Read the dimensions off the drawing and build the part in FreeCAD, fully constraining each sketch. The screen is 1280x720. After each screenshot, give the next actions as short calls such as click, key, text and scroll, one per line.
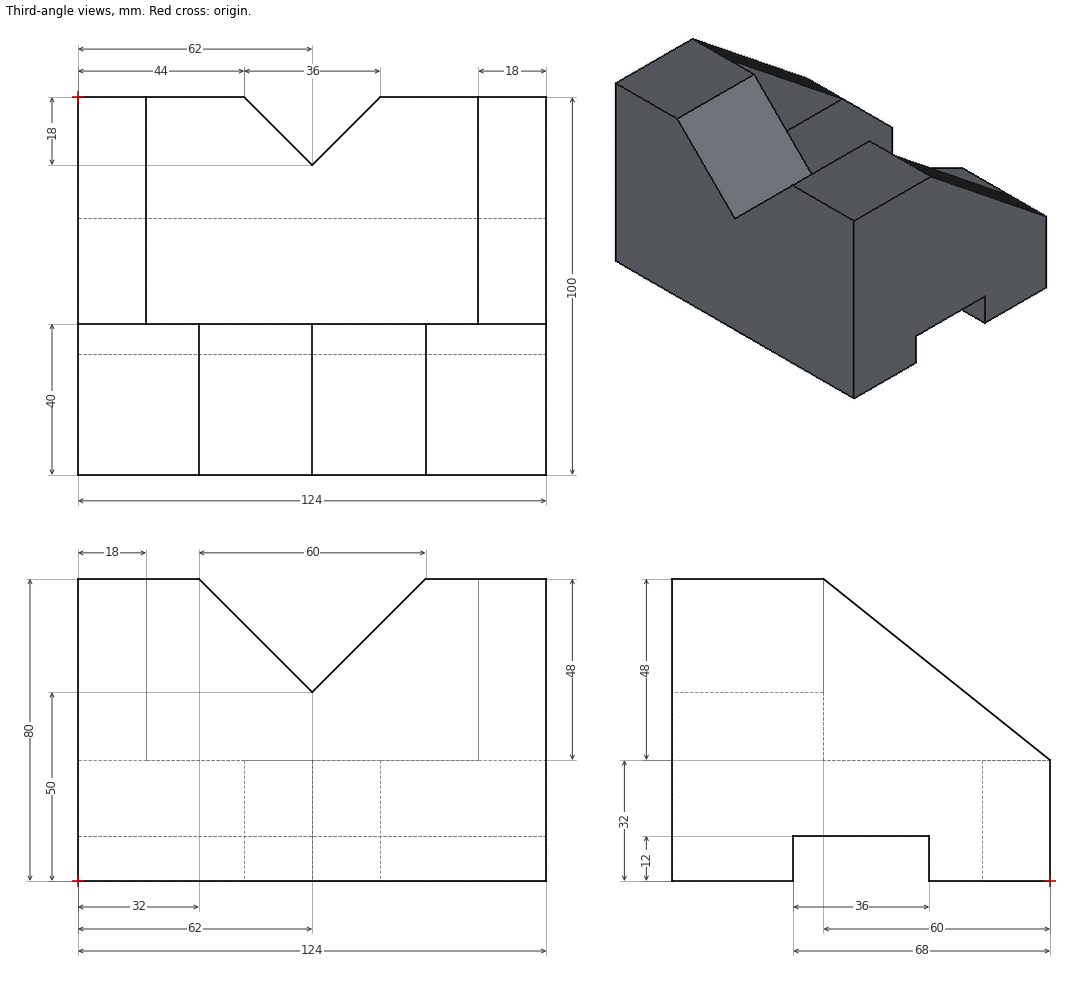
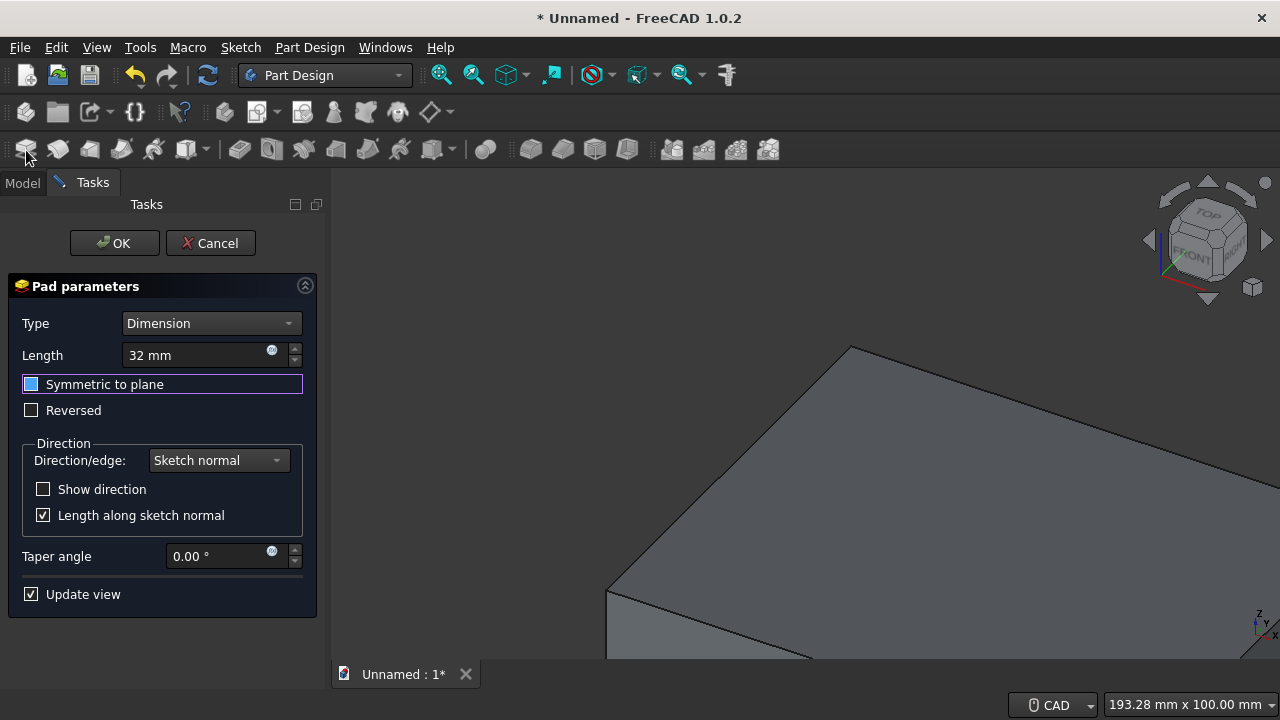
click(115, 243)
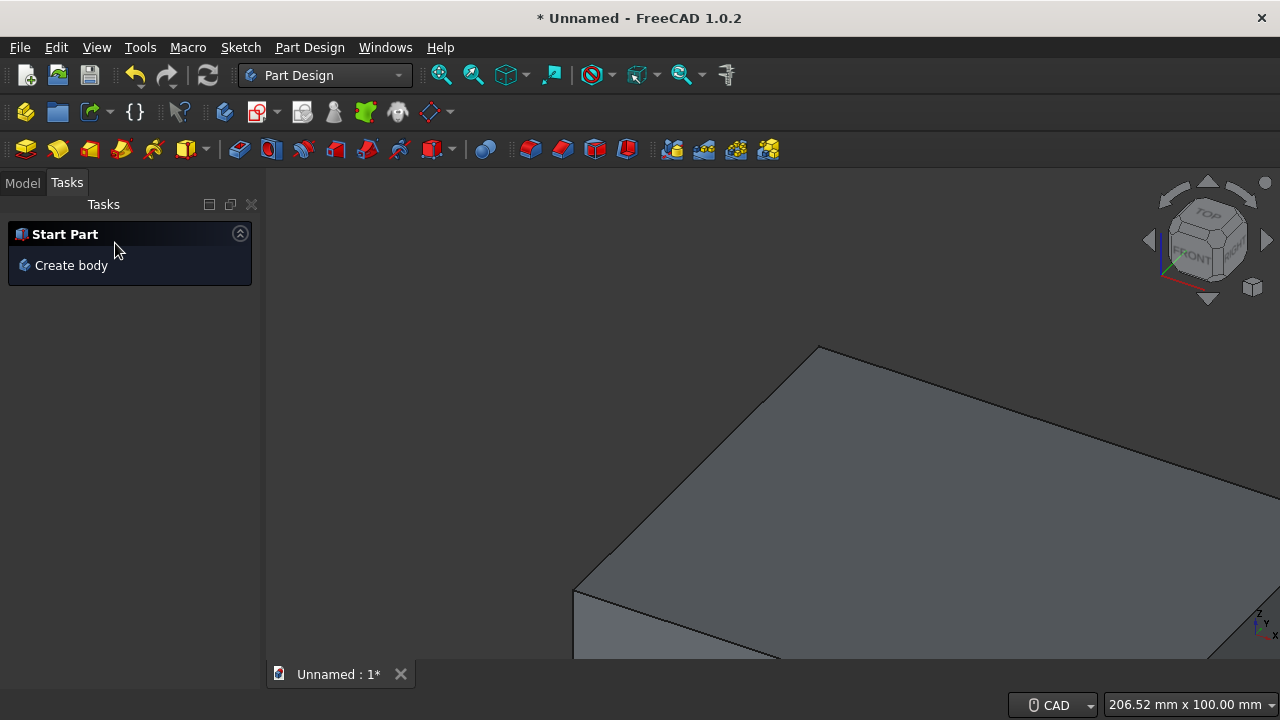
click(442, 76)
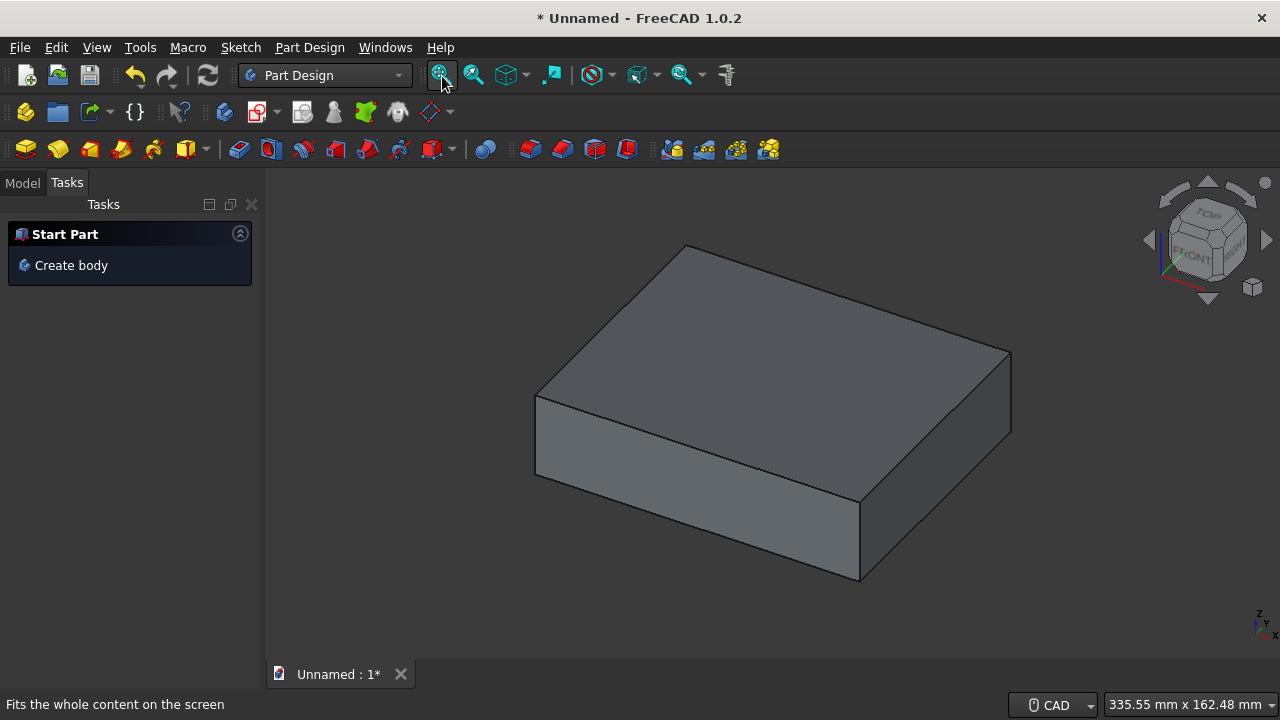
click(258, 112)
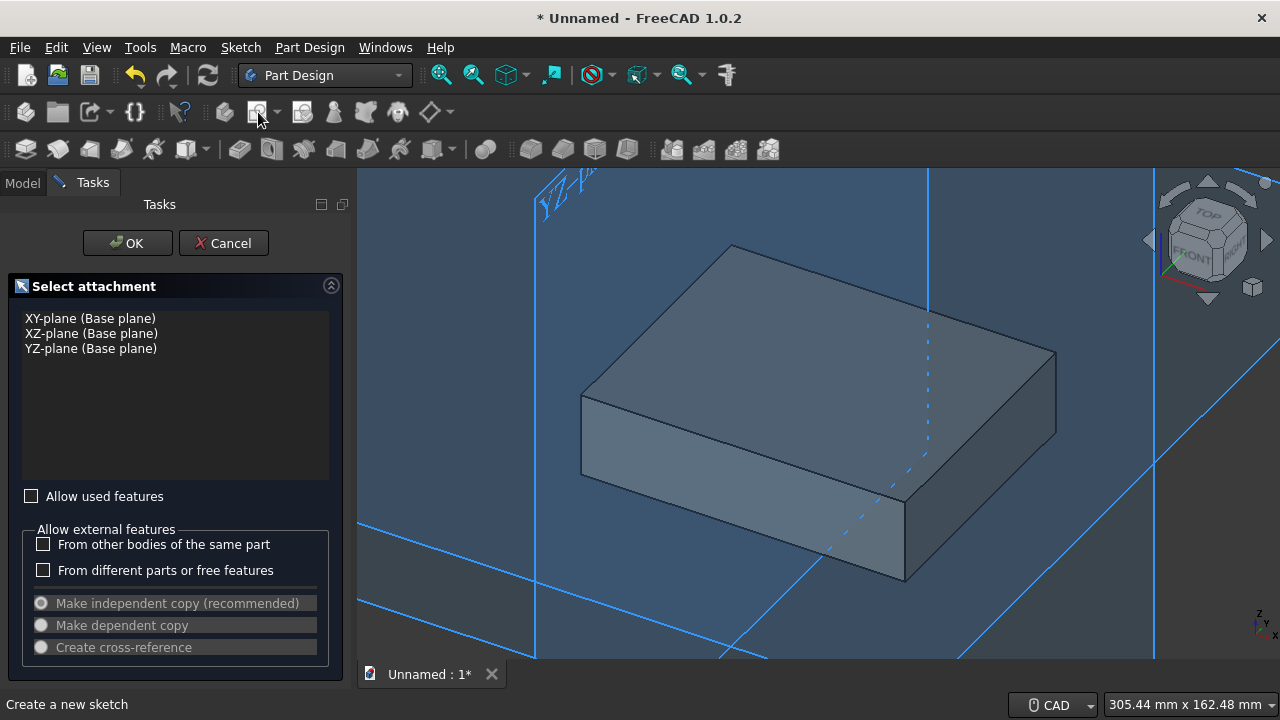
click(82, 348)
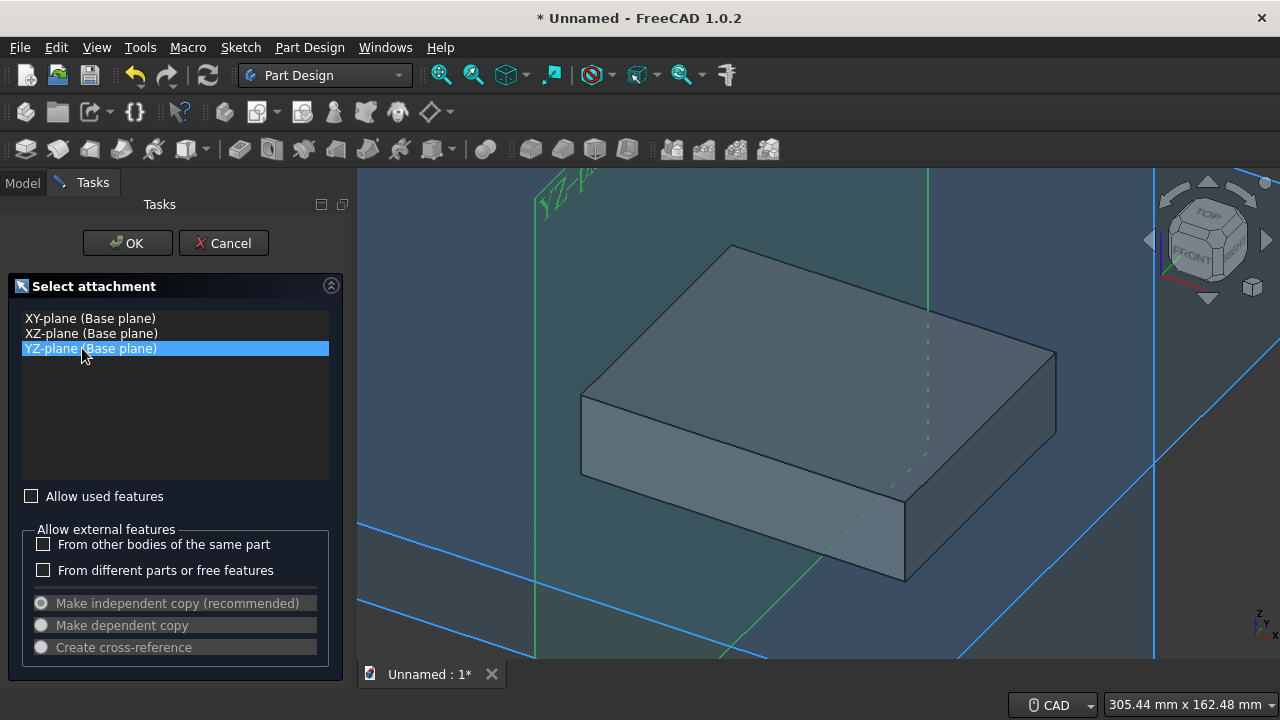
click(128, 243)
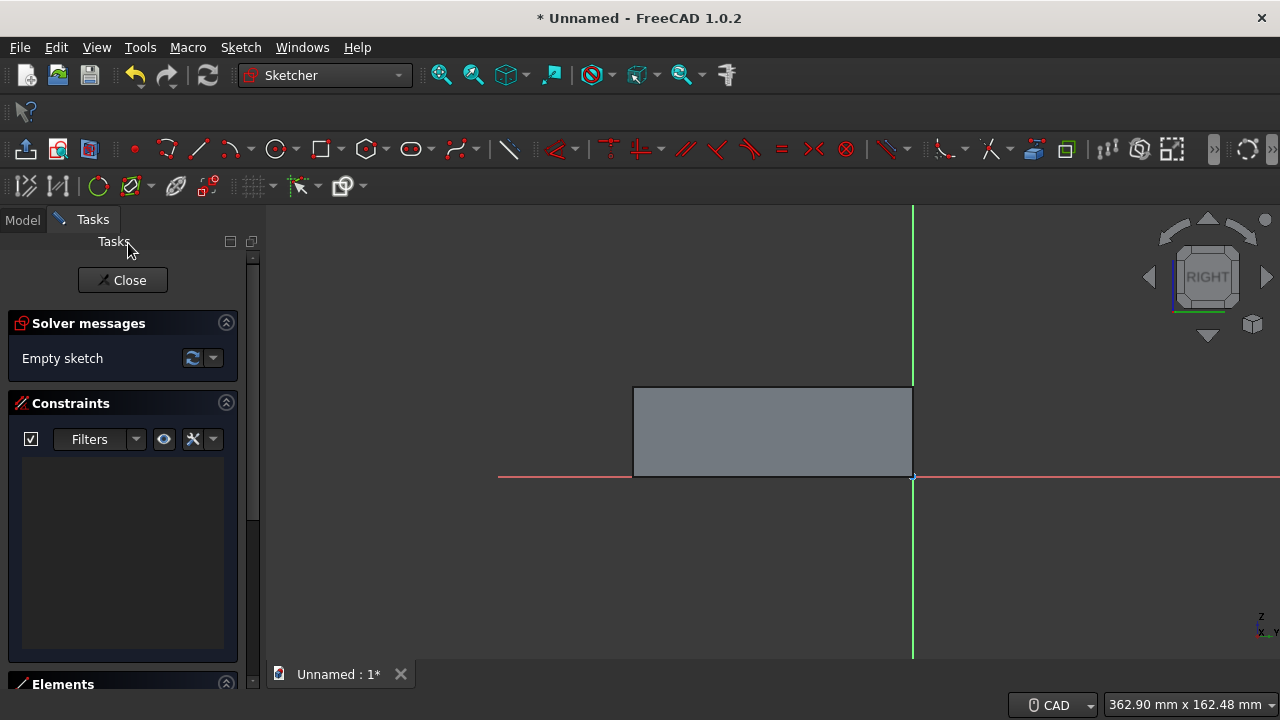
click(90, 150)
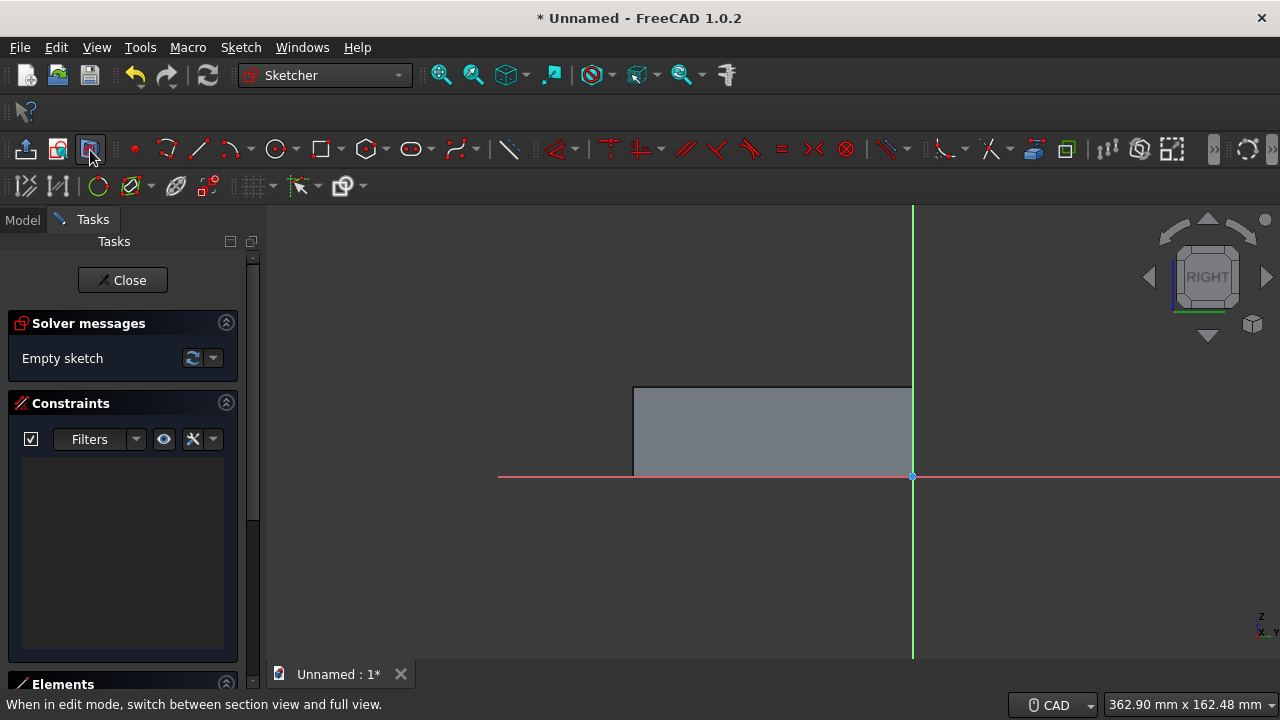
scroll(867, 472, up, 6)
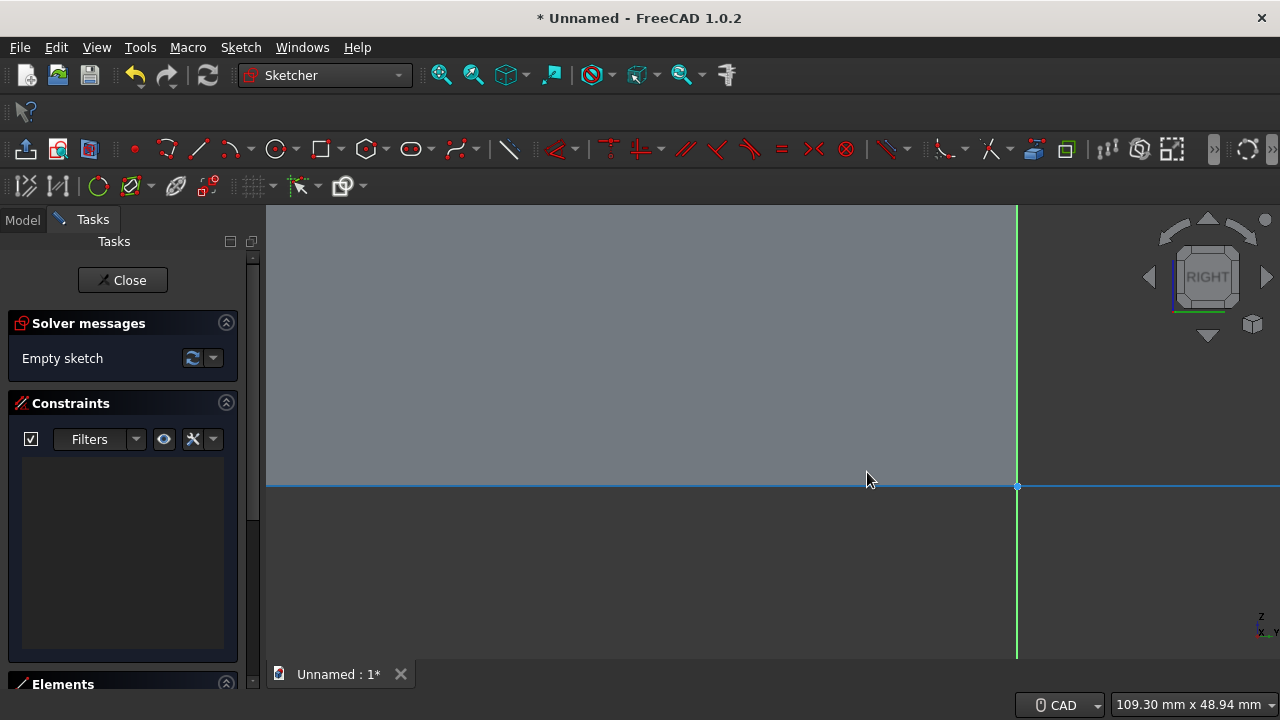
click(322, 150)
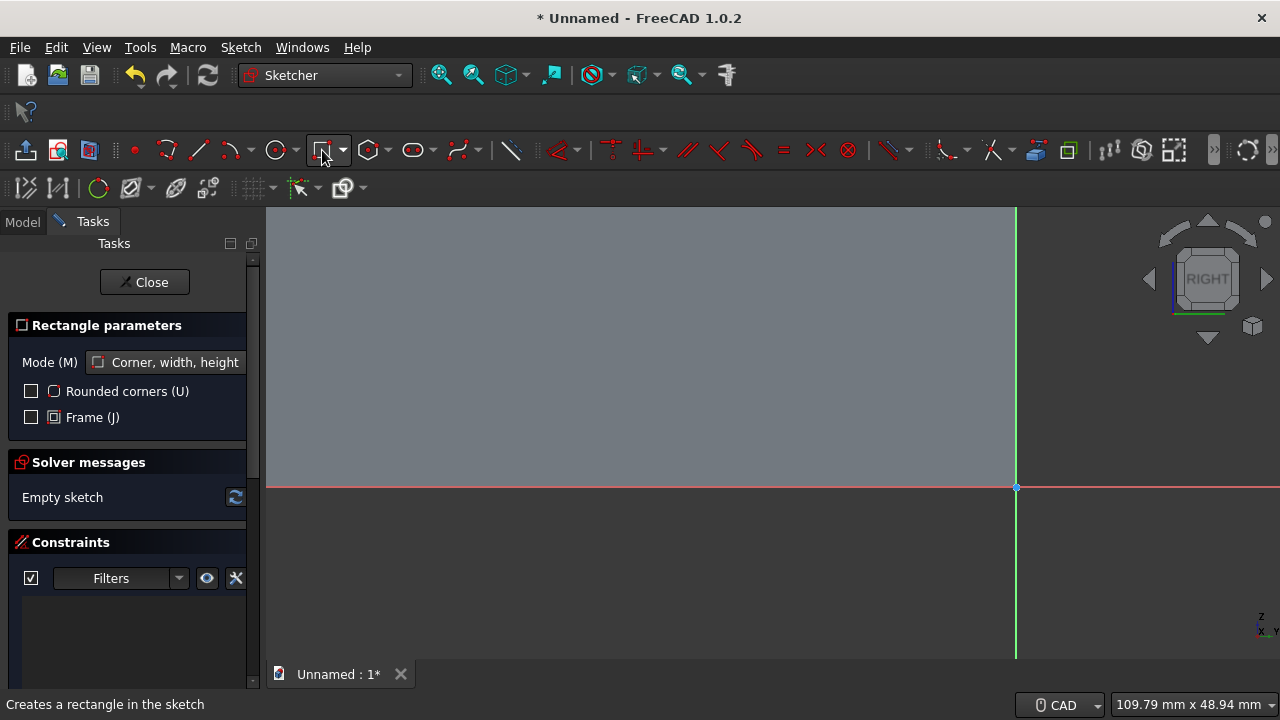
click(388, 376)
click(721, 487)
key(Escape)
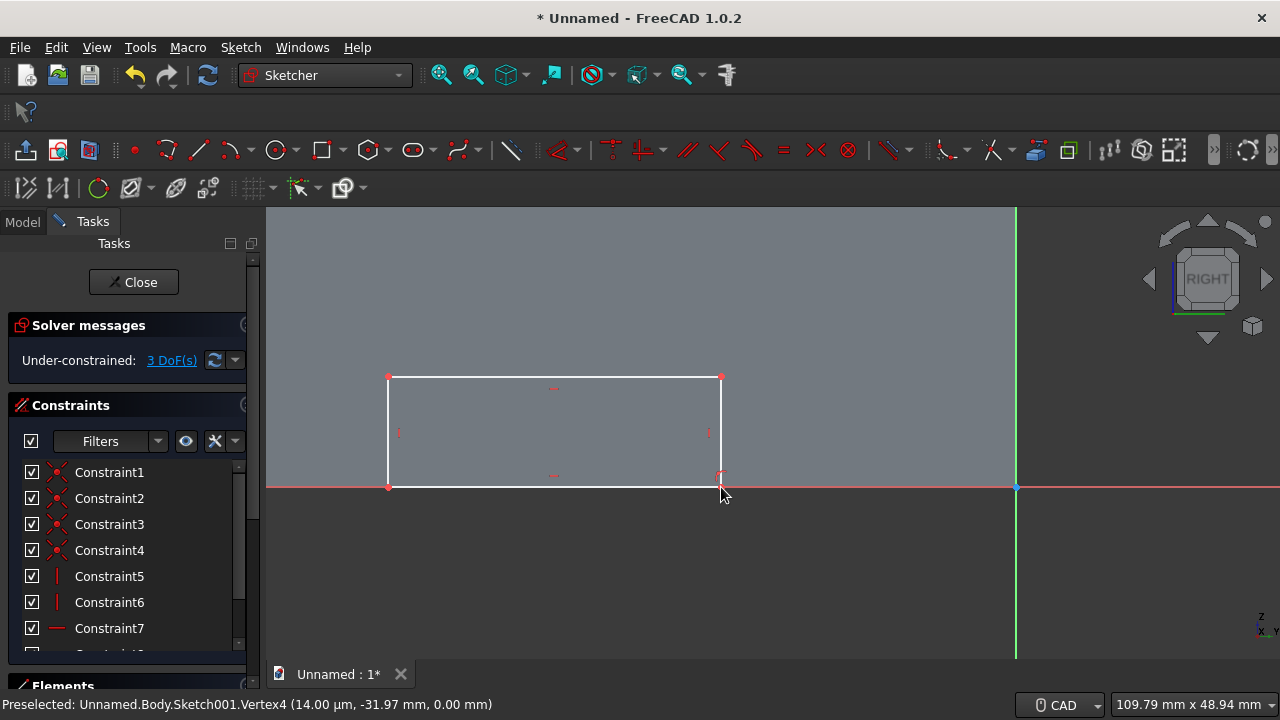
click(558, 150)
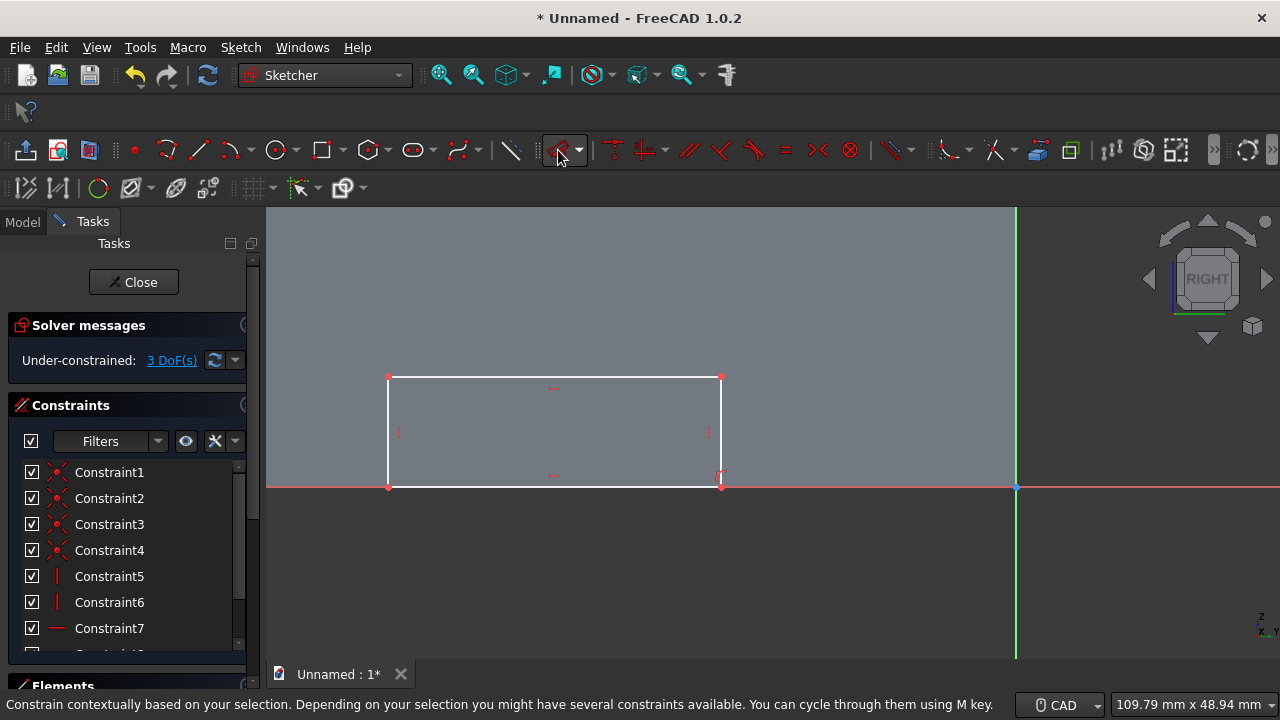
click(388, 410)
click(354, 432)